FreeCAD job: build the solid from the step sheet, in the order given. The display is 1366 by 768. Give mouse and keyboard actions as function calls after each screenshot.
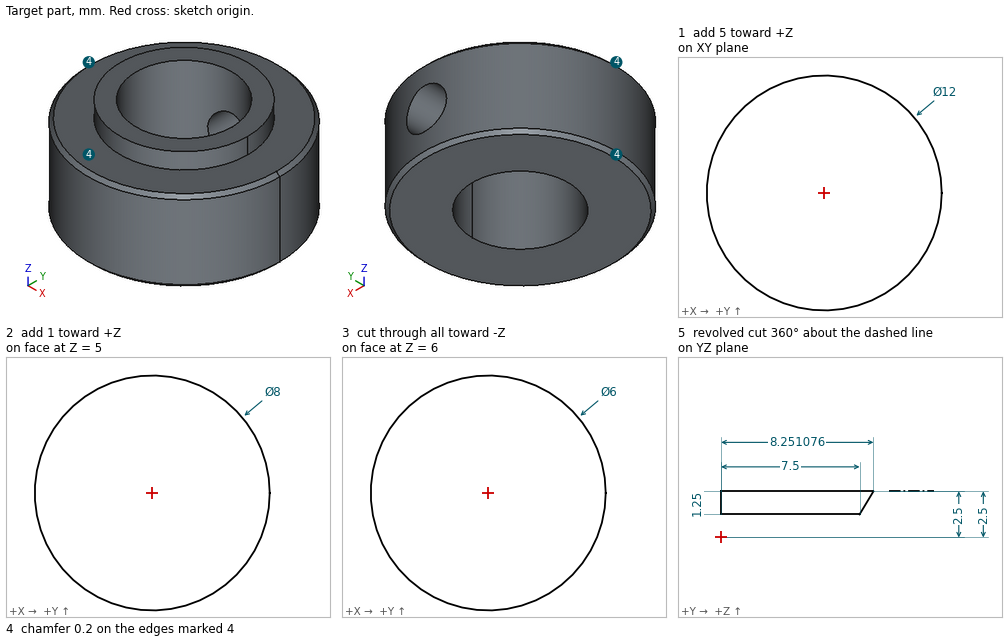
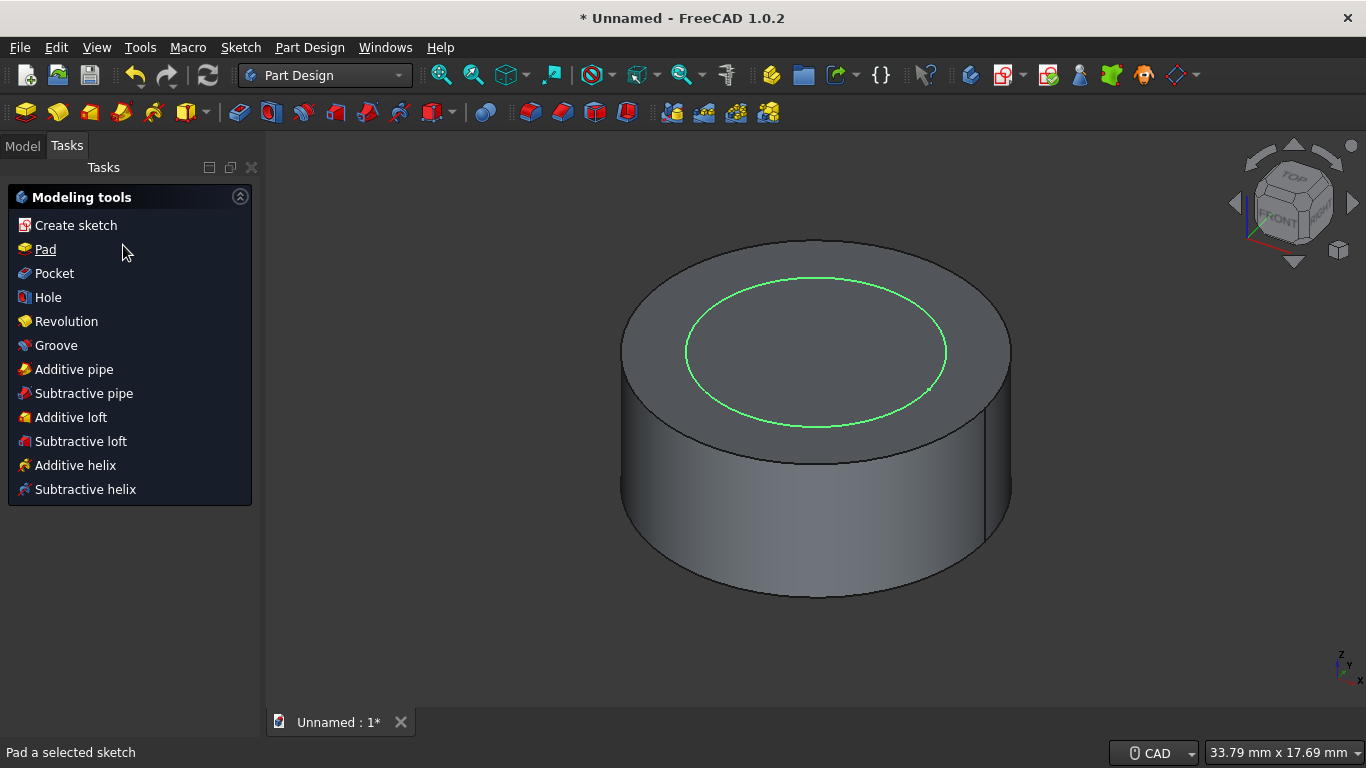
click(26, 112)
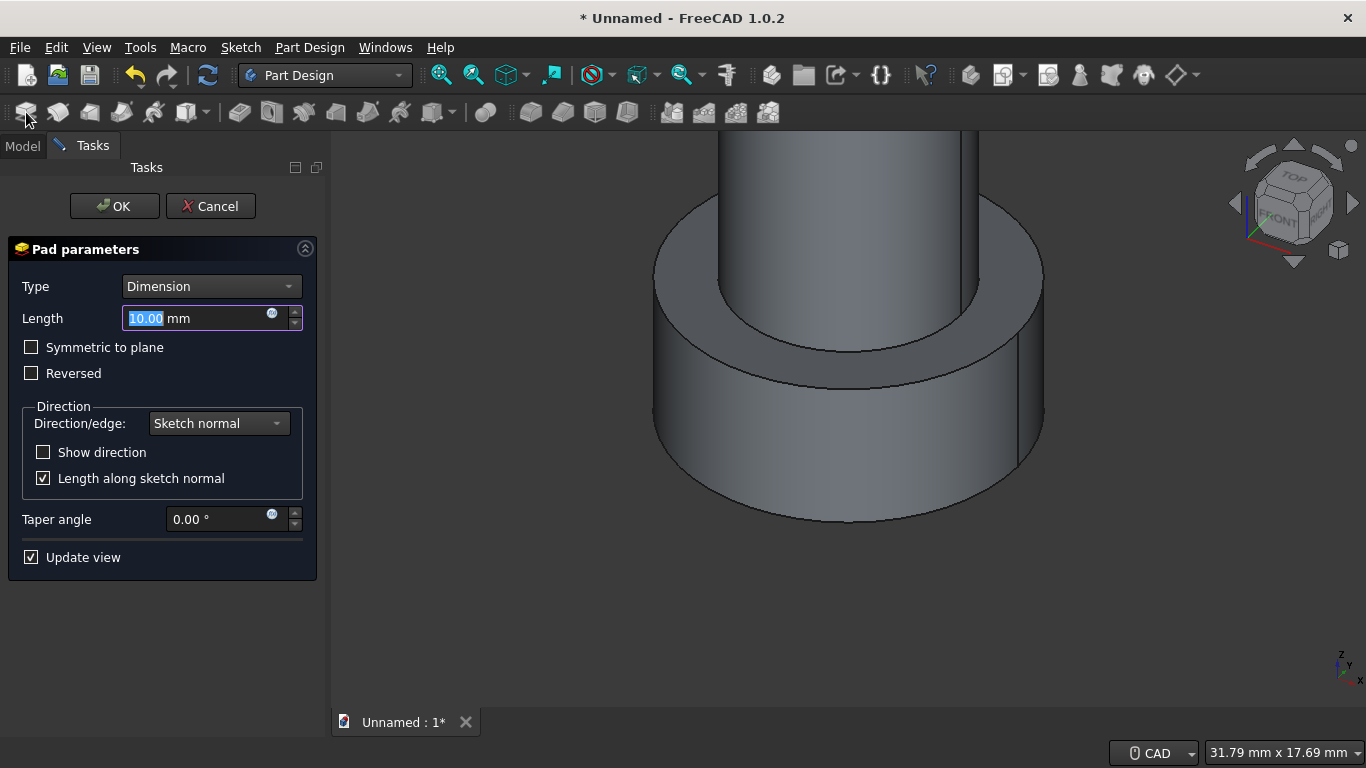
text(1)
key(Tab)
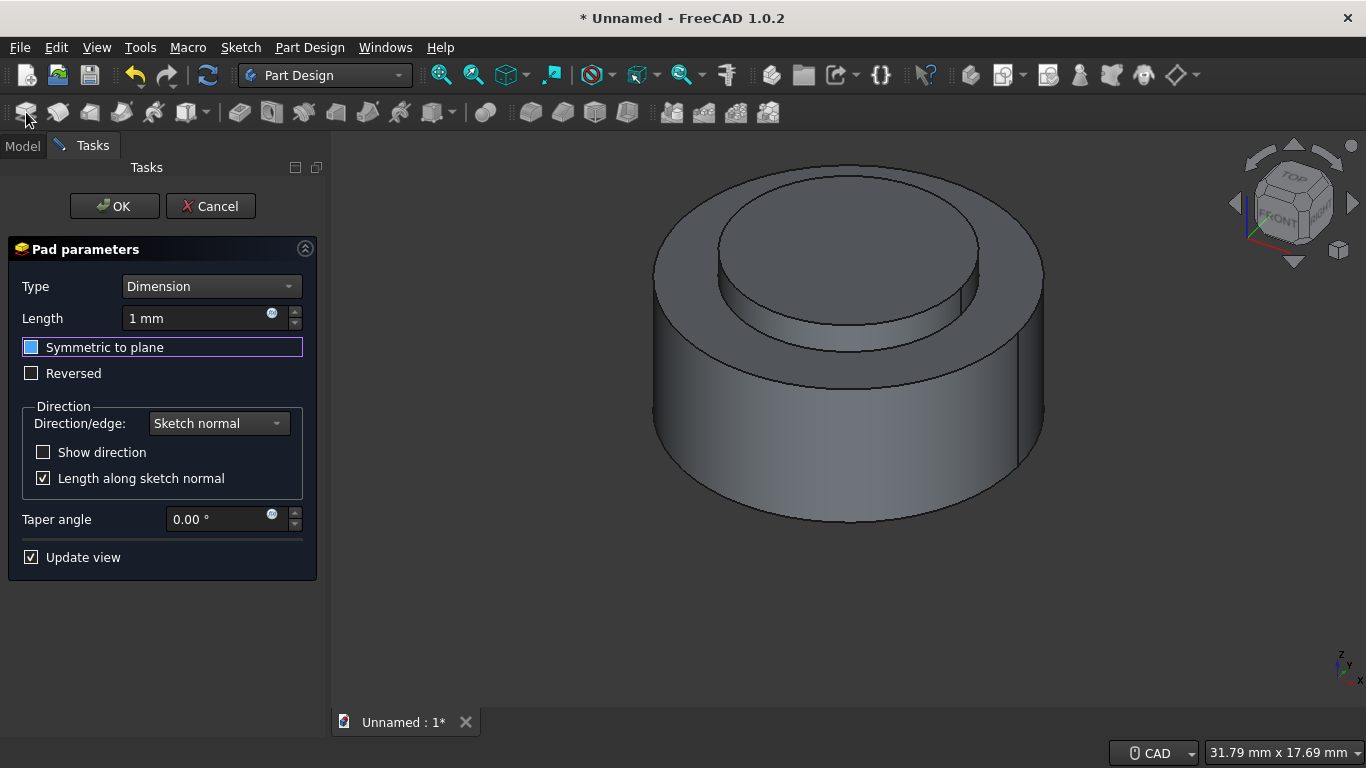
click(115, 206)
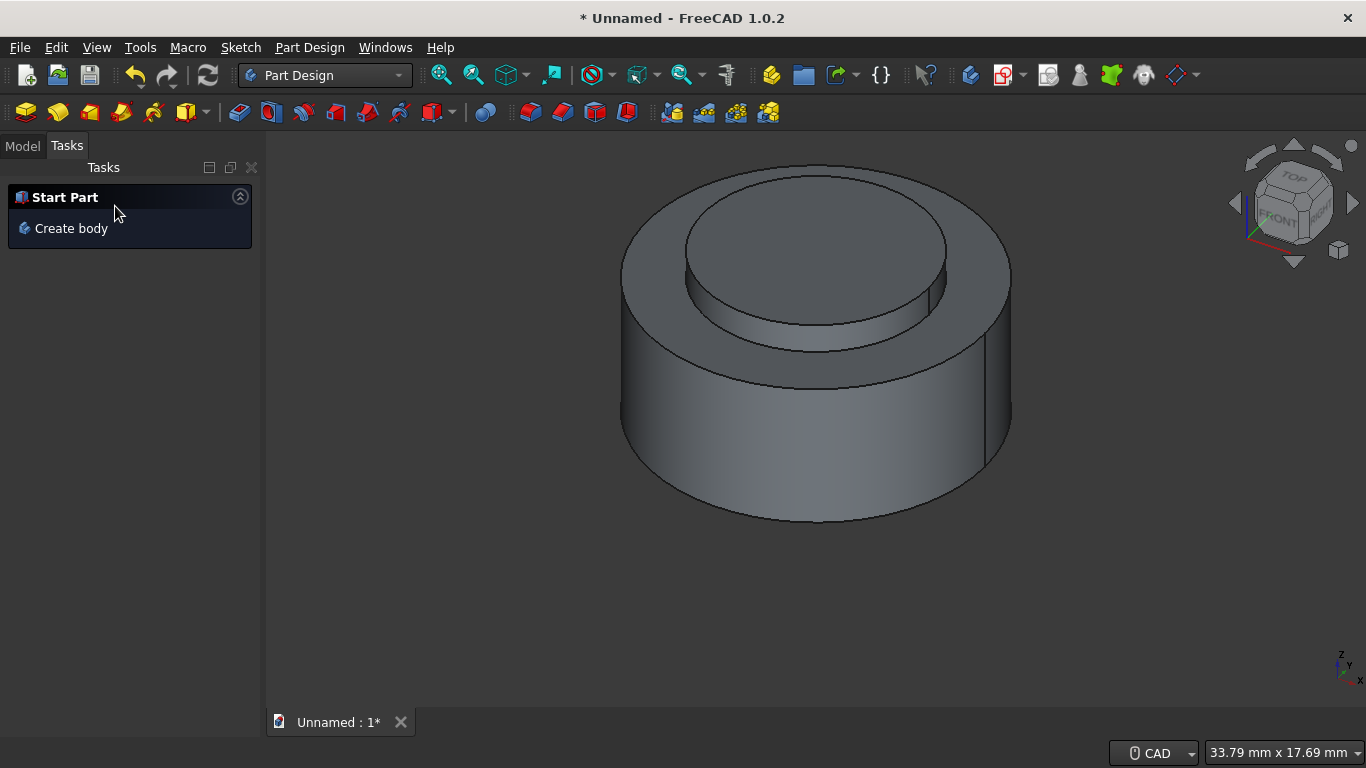
click(442, 76)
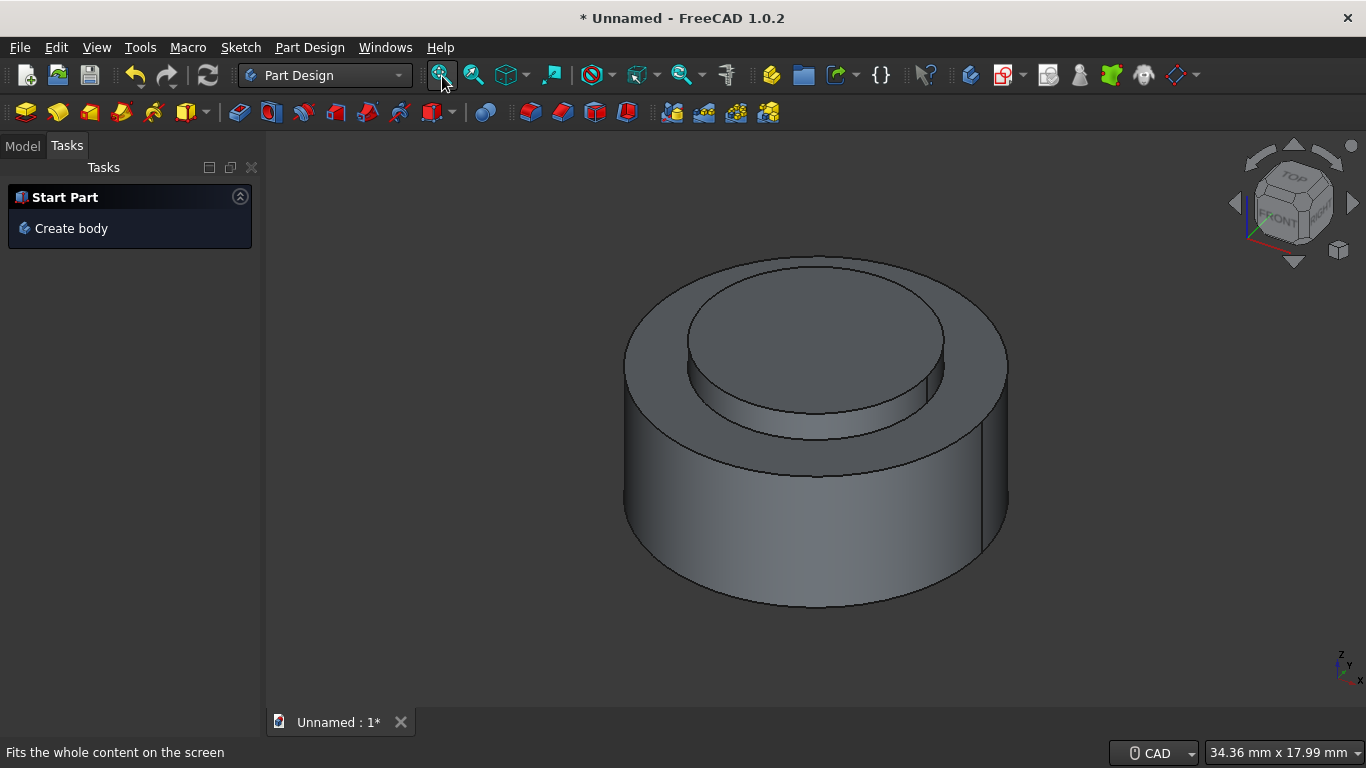
click(816, 339)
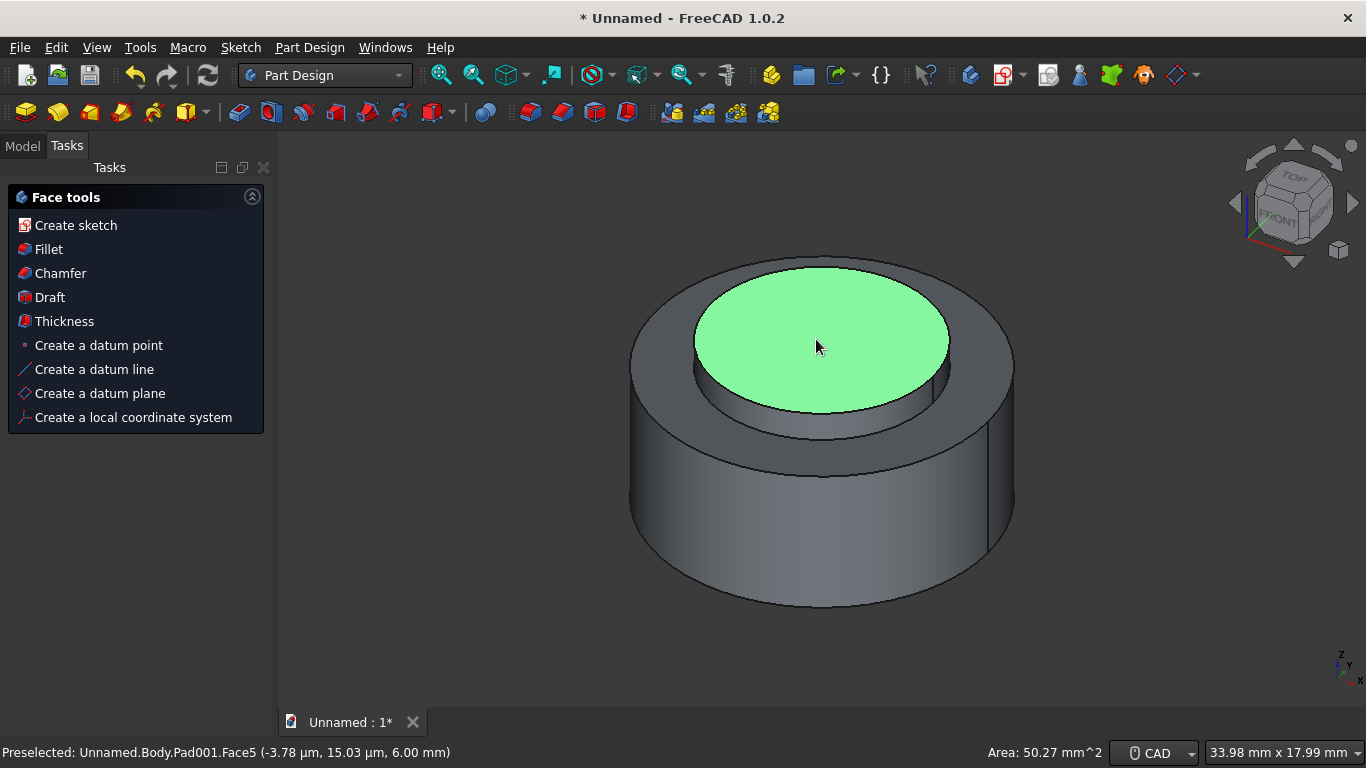
click(1004, 76)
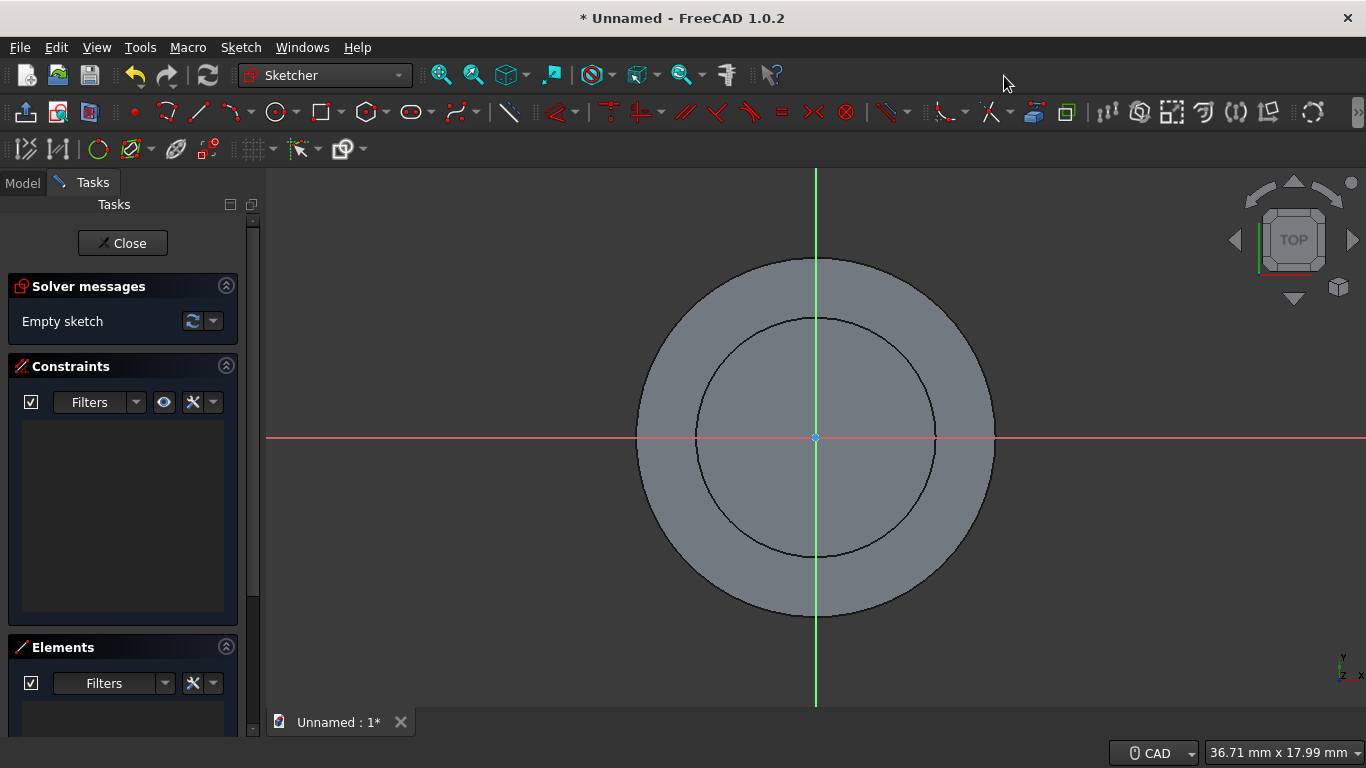
scroll(899, 438, up, 3)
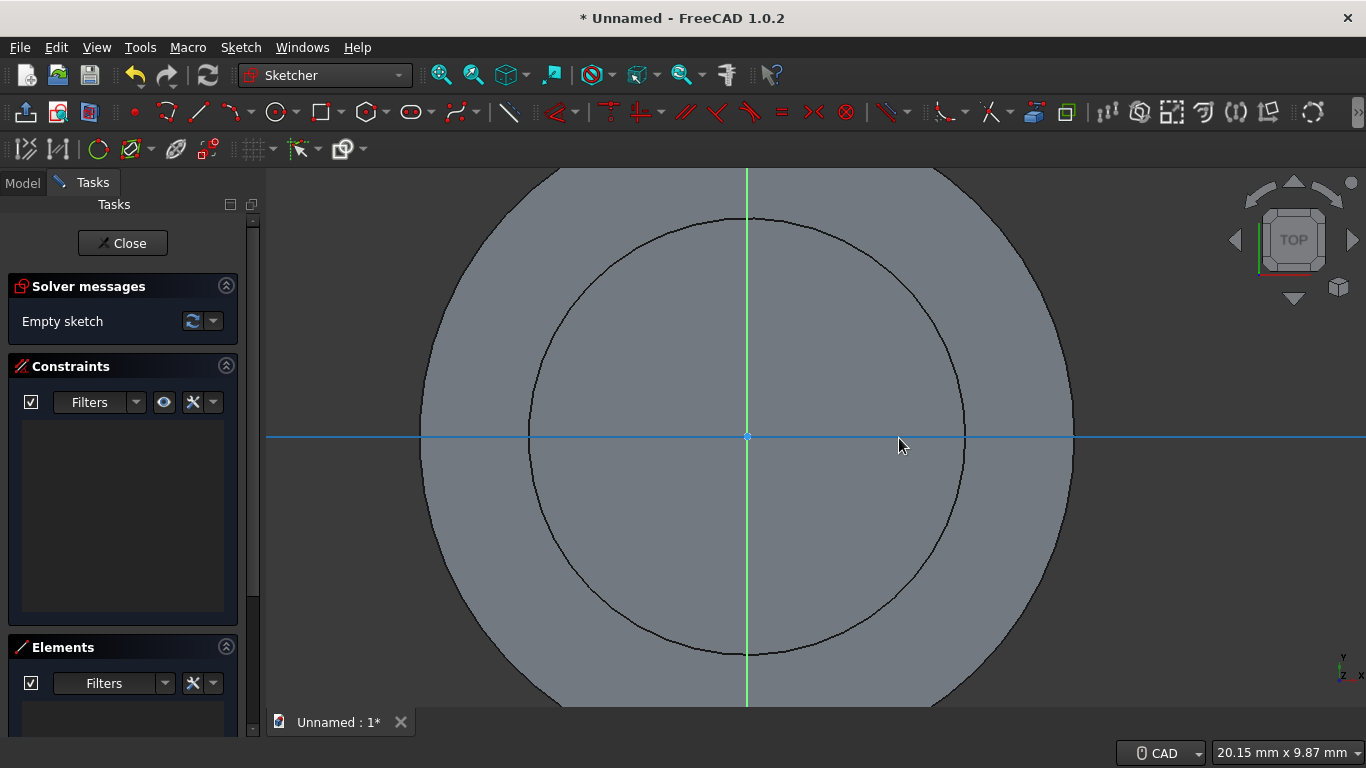
click(276, 112)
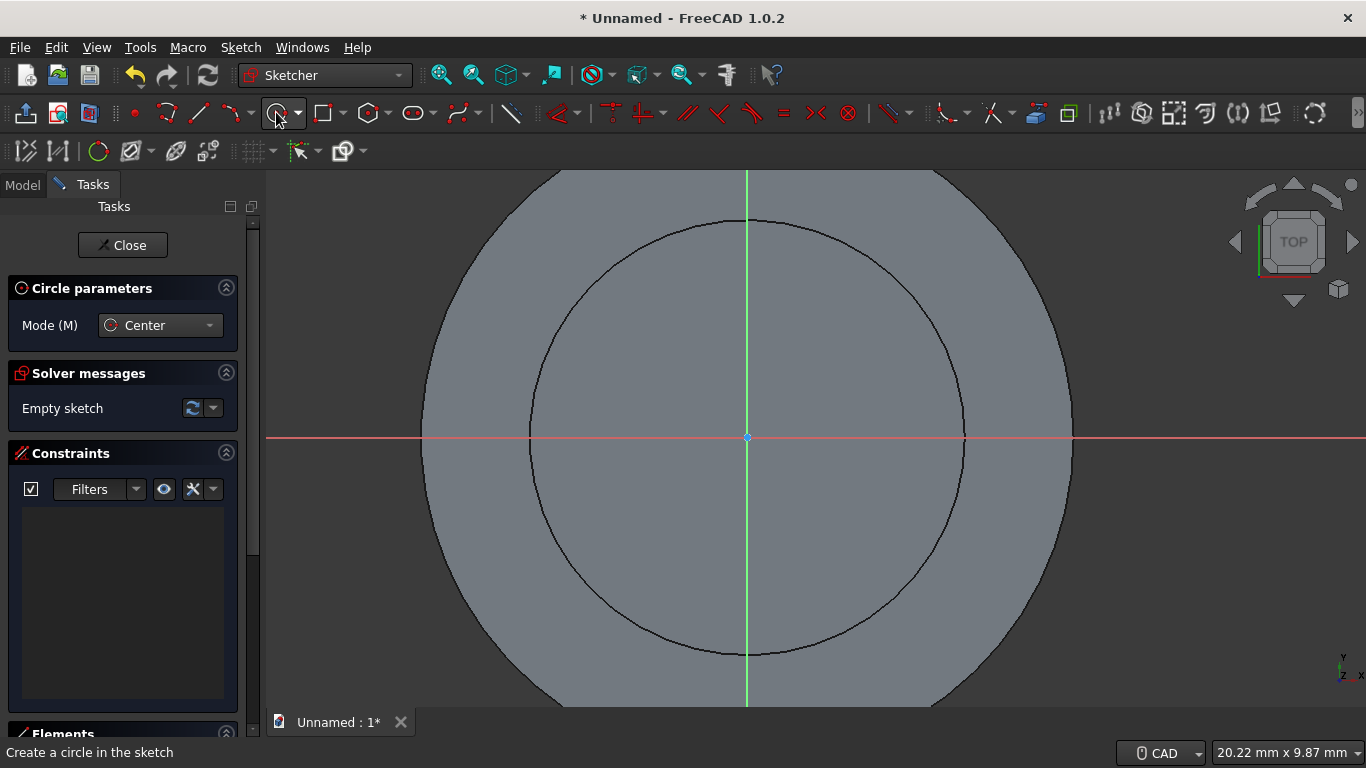
click(747, 438)
move(863, 322)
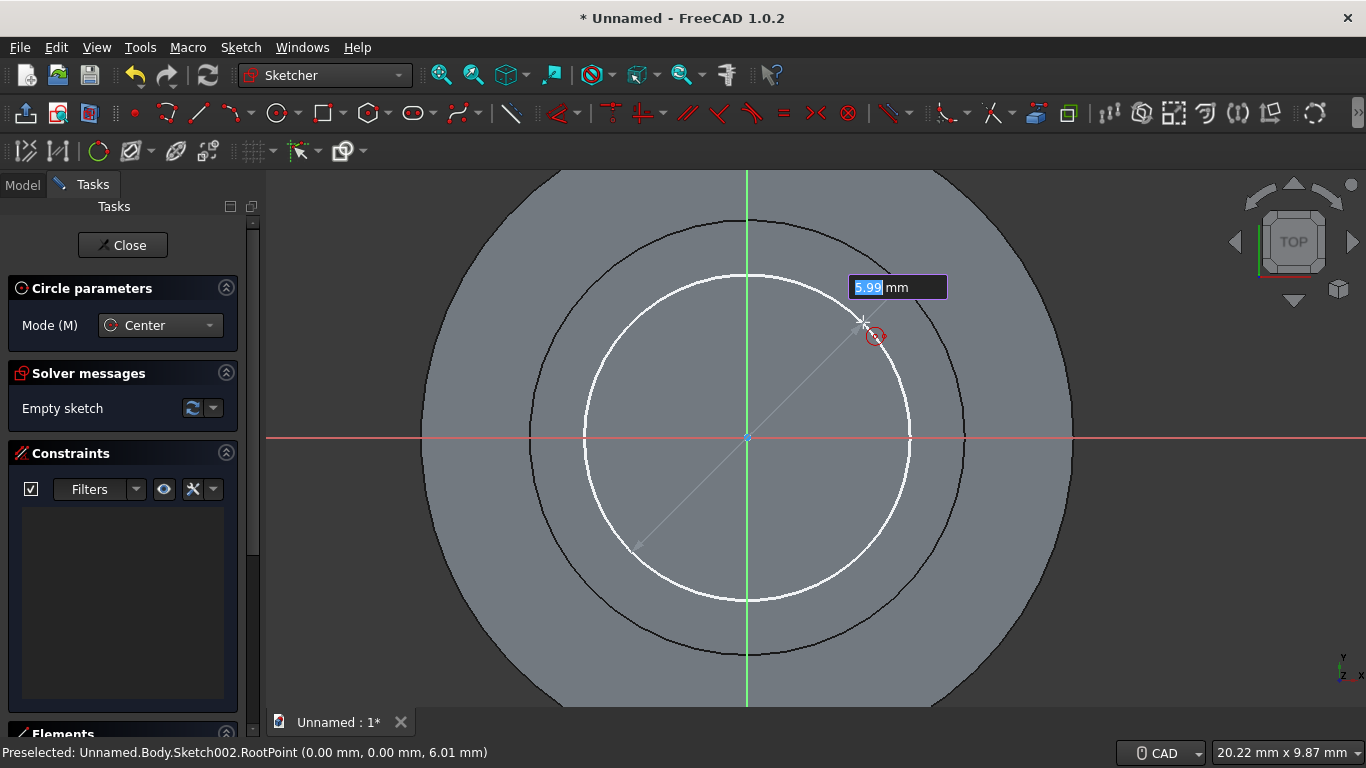
text(6)
key(Return)
key(Escape)